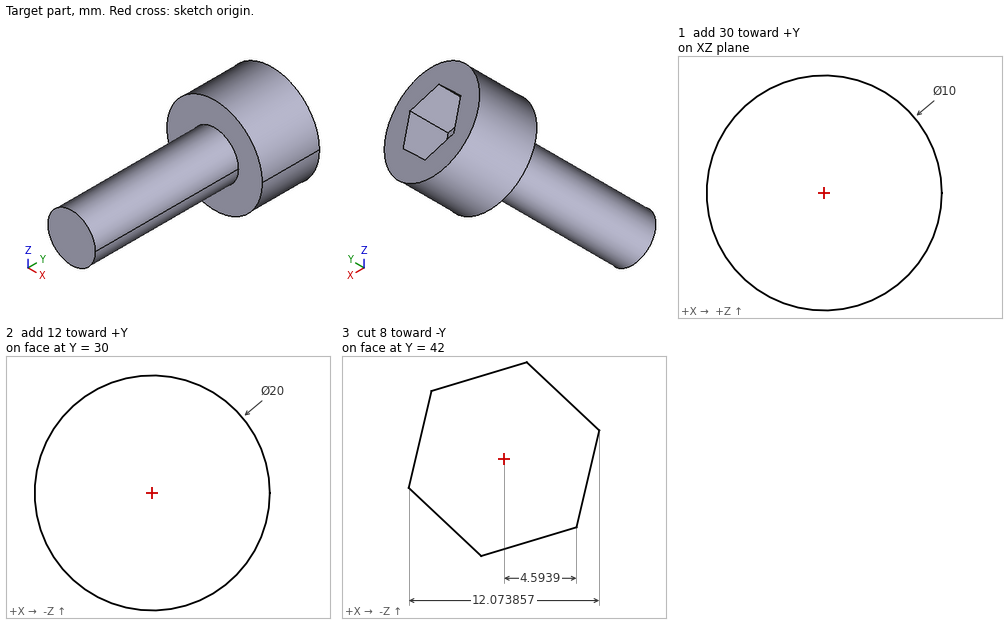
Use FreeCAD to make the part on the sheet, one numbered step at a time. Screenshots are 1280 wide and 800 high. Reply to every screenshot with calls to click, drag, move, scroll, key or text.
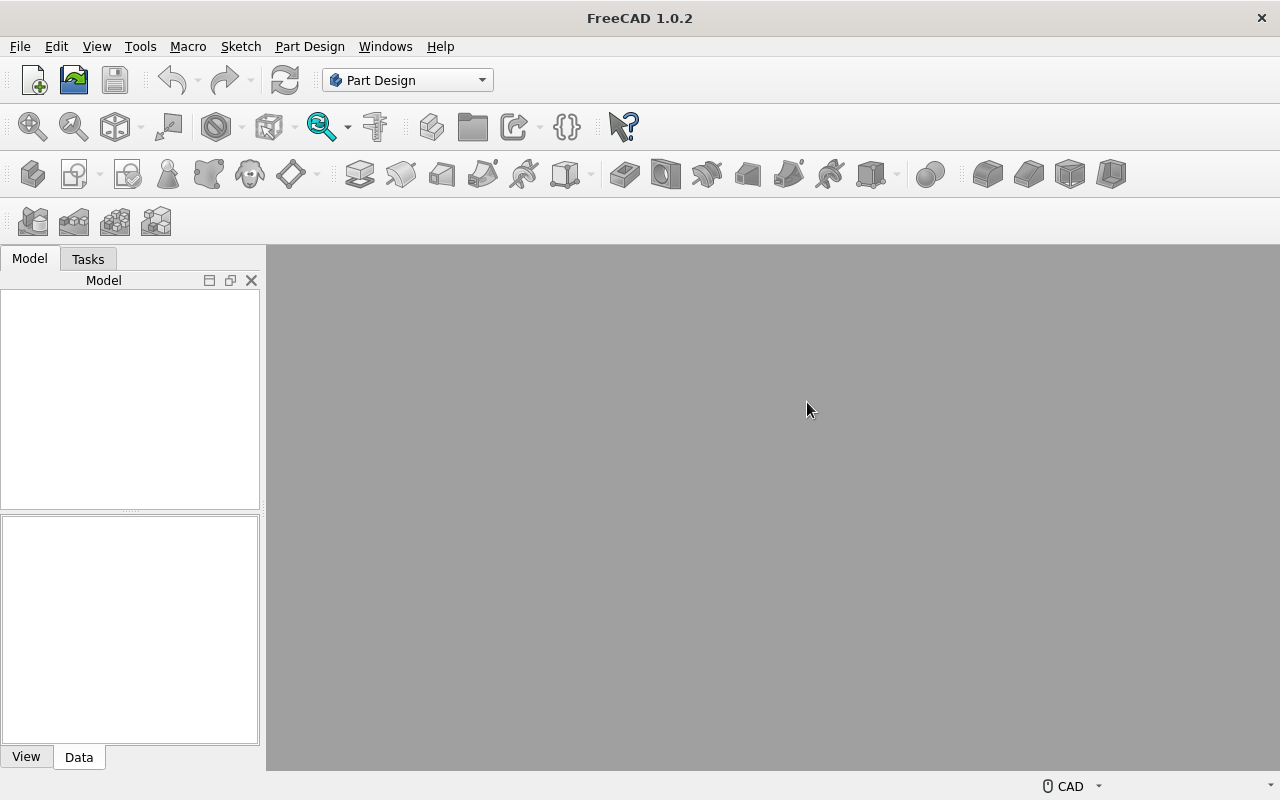
click(33, 80)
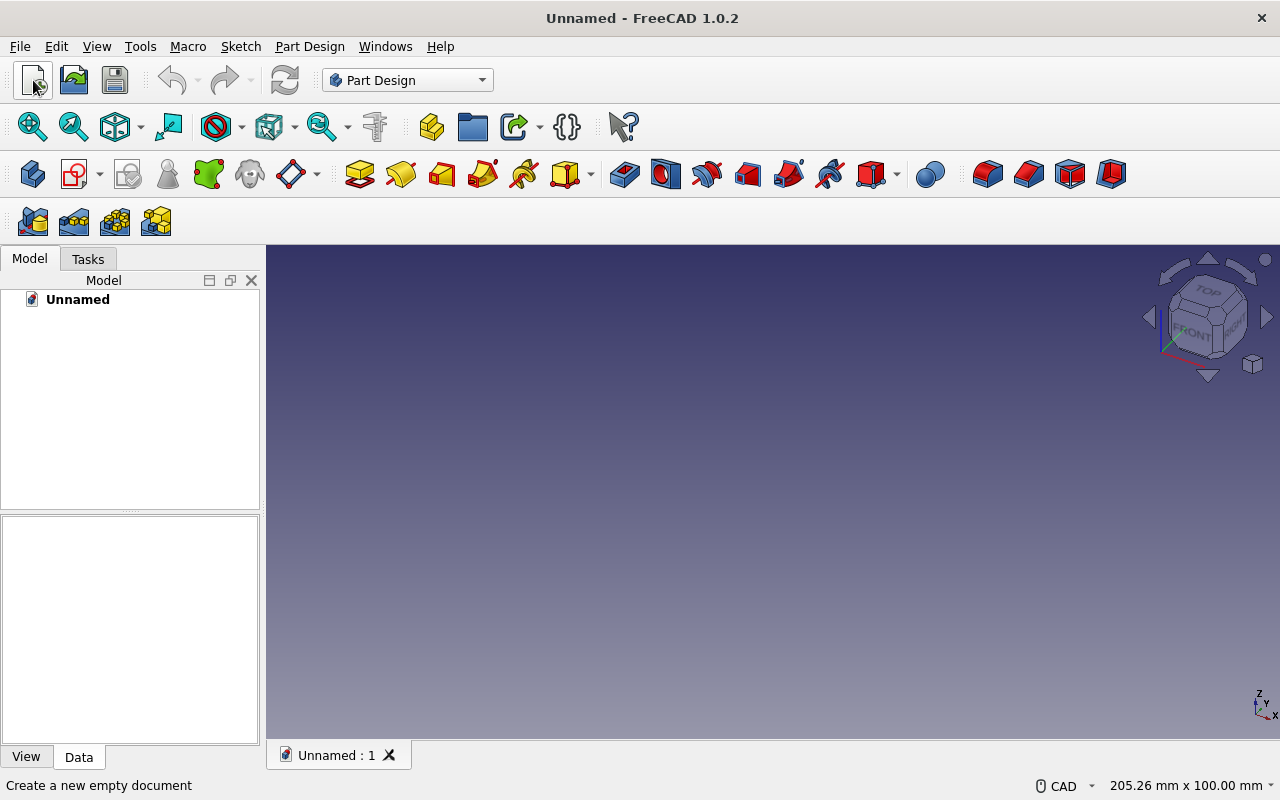
click(74, 174)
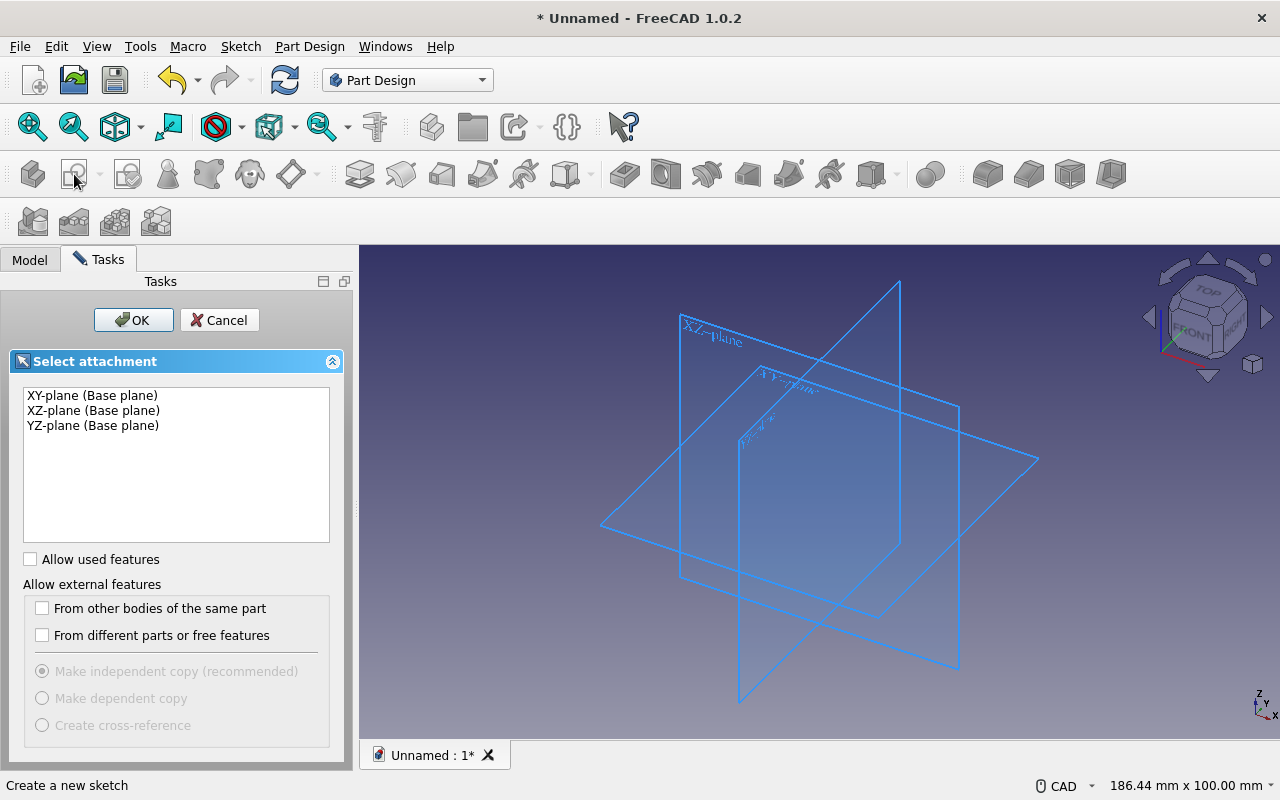
click(84, 410)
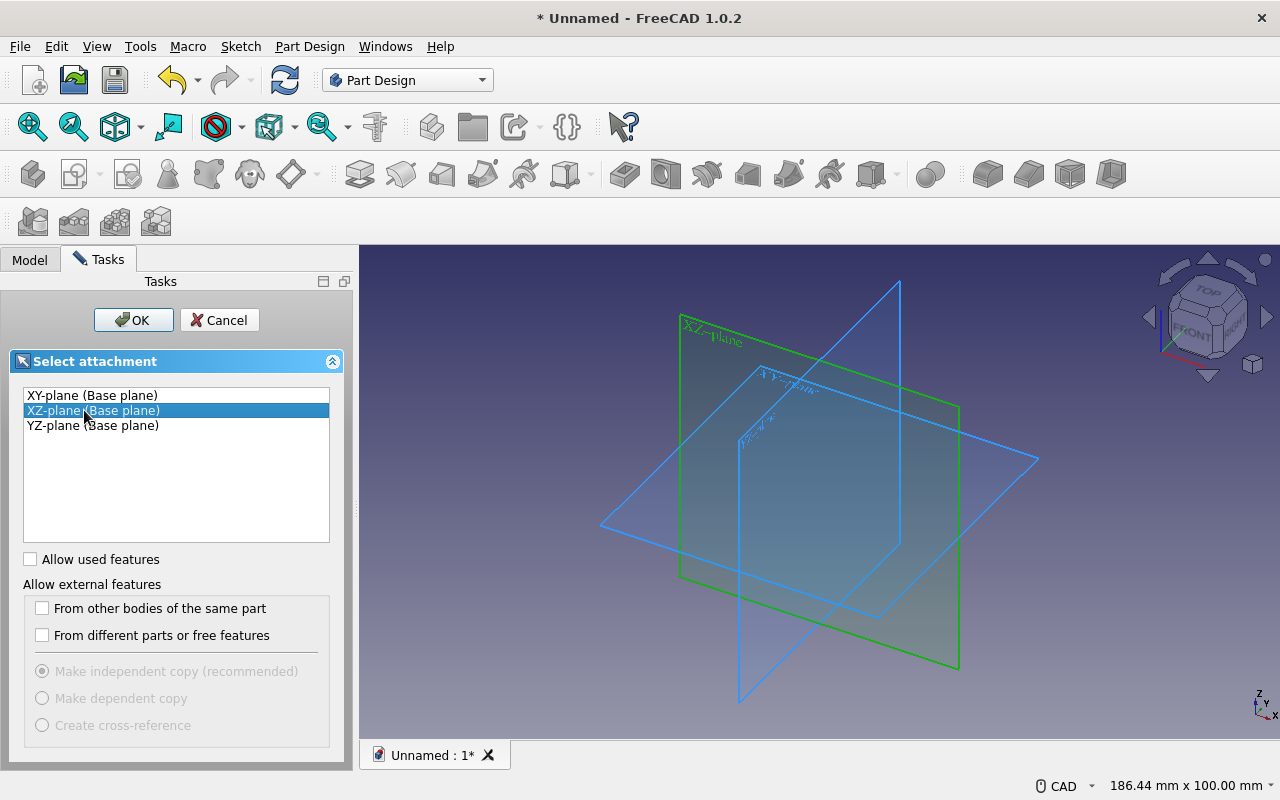
click(134, 320)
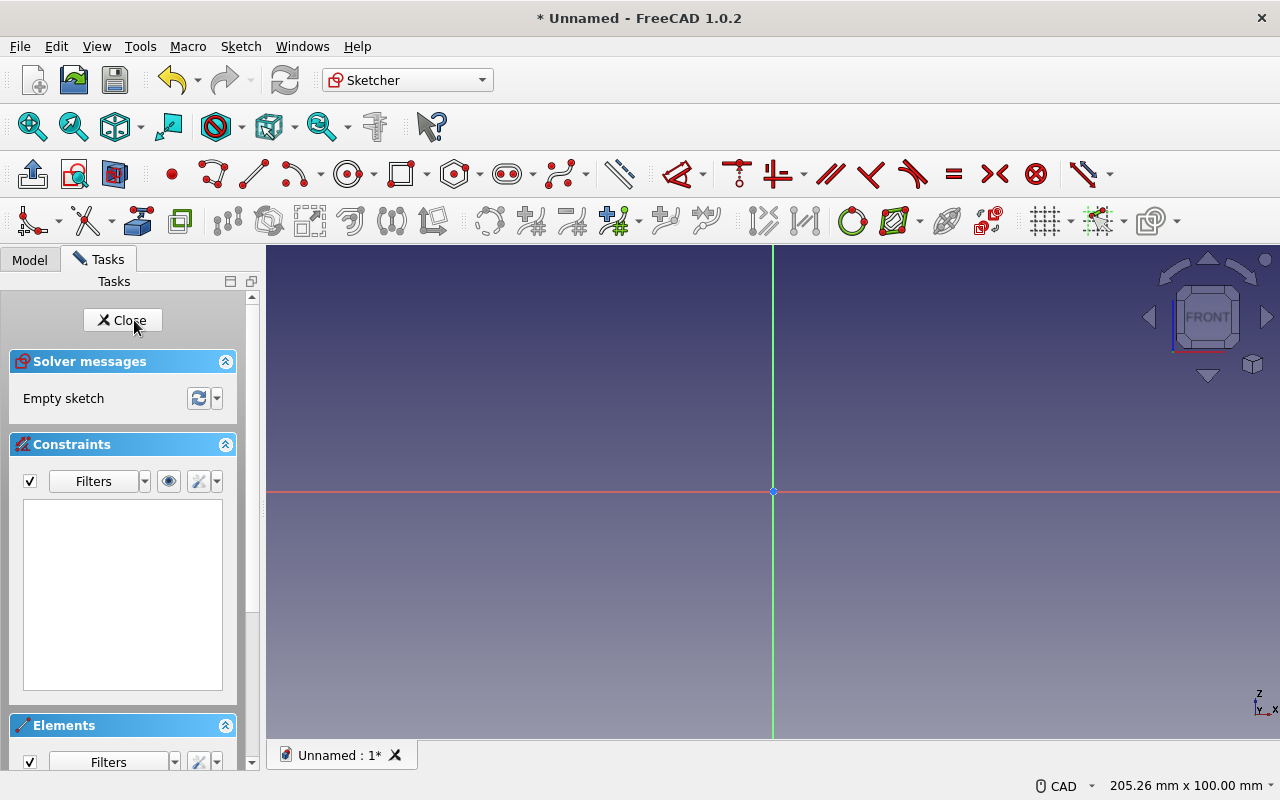
scroll(787, 492, up, 9)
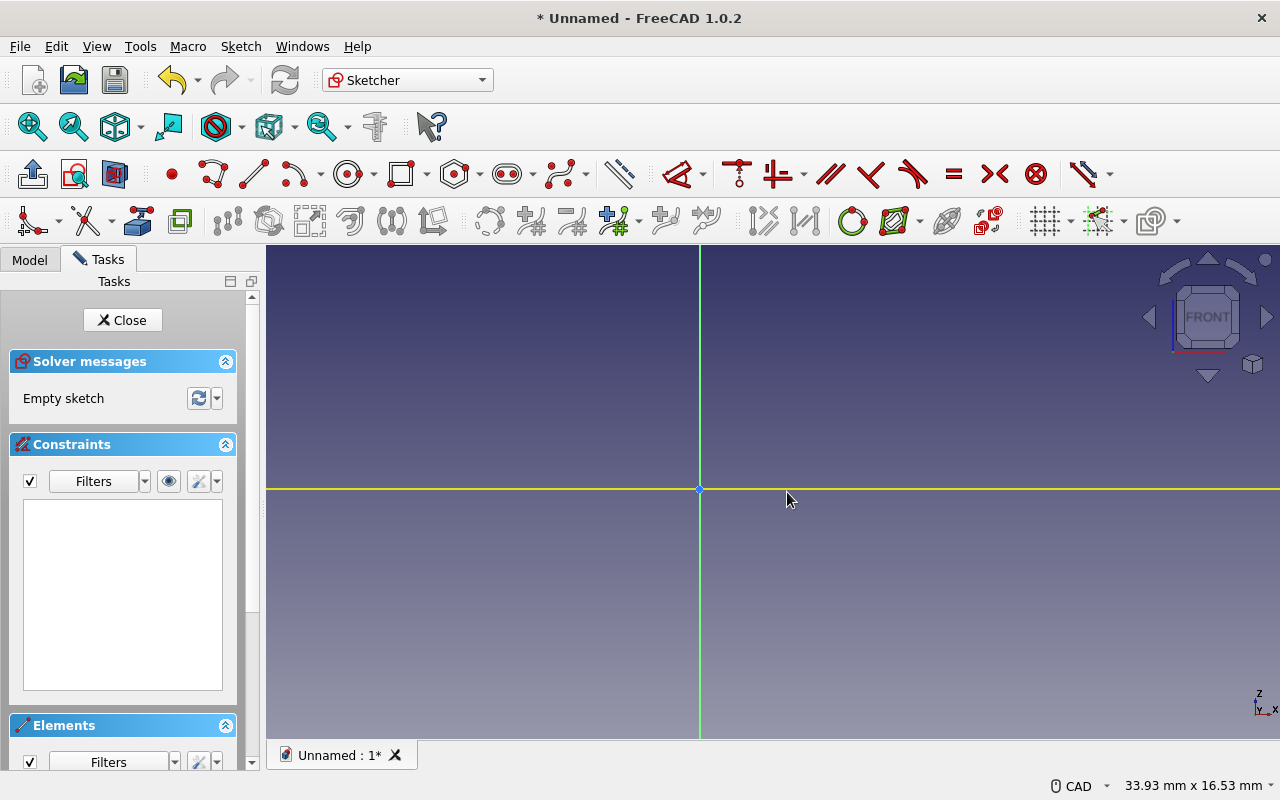
click(348, 174)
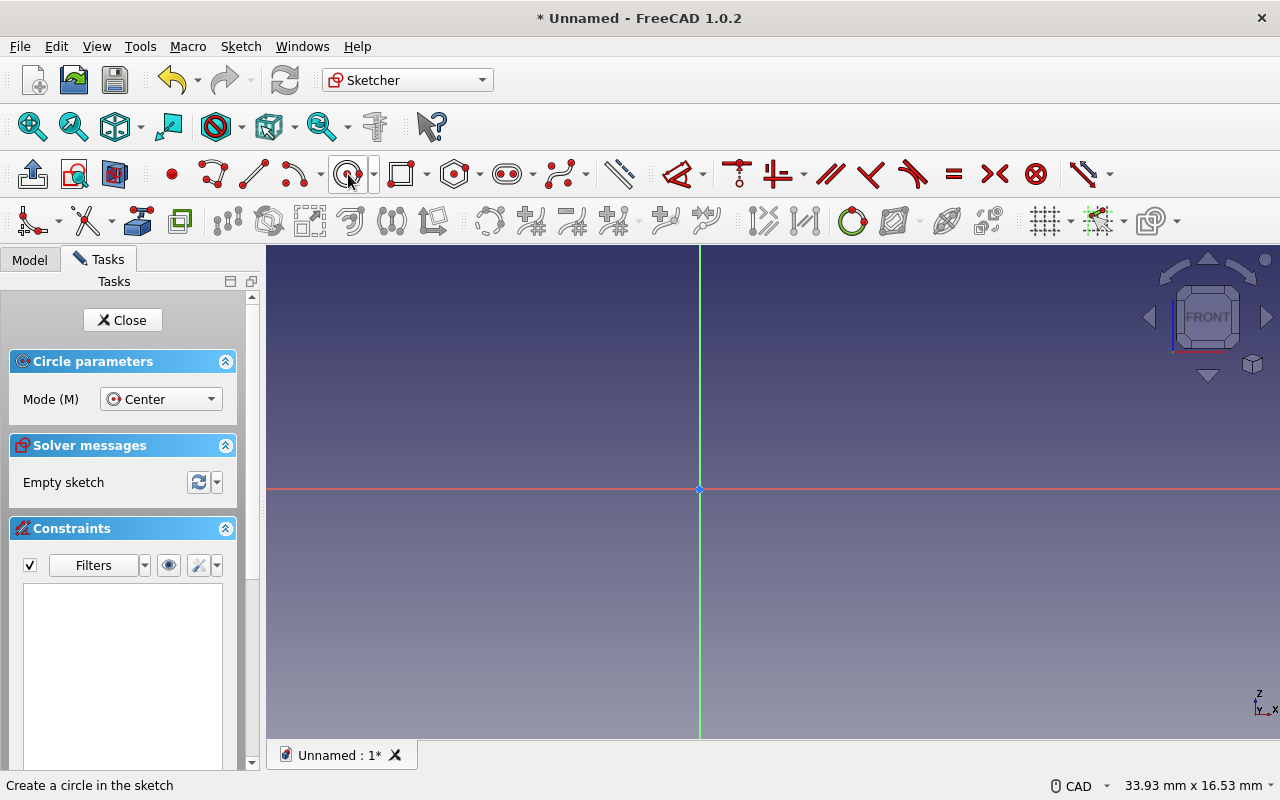
click(700, 489)
move(805, 384)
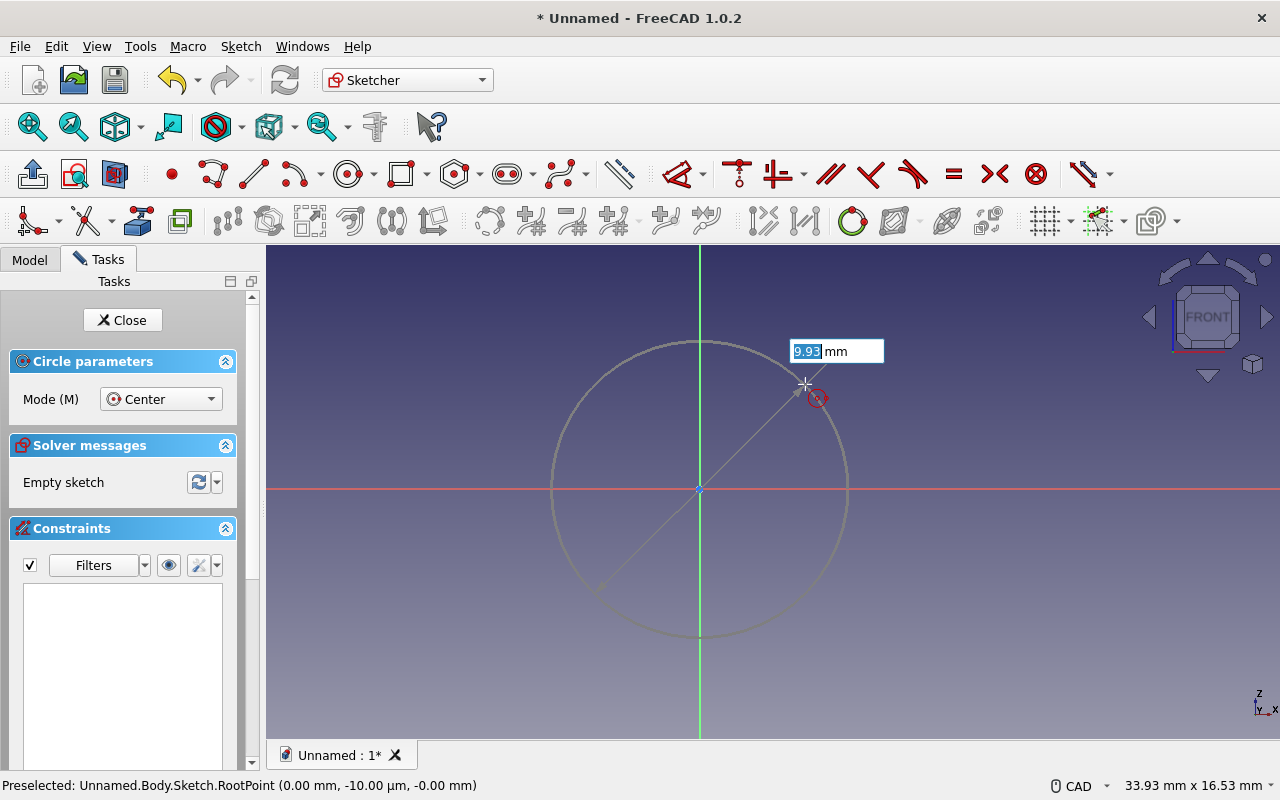
text(10)
key(Return)
key(Escape)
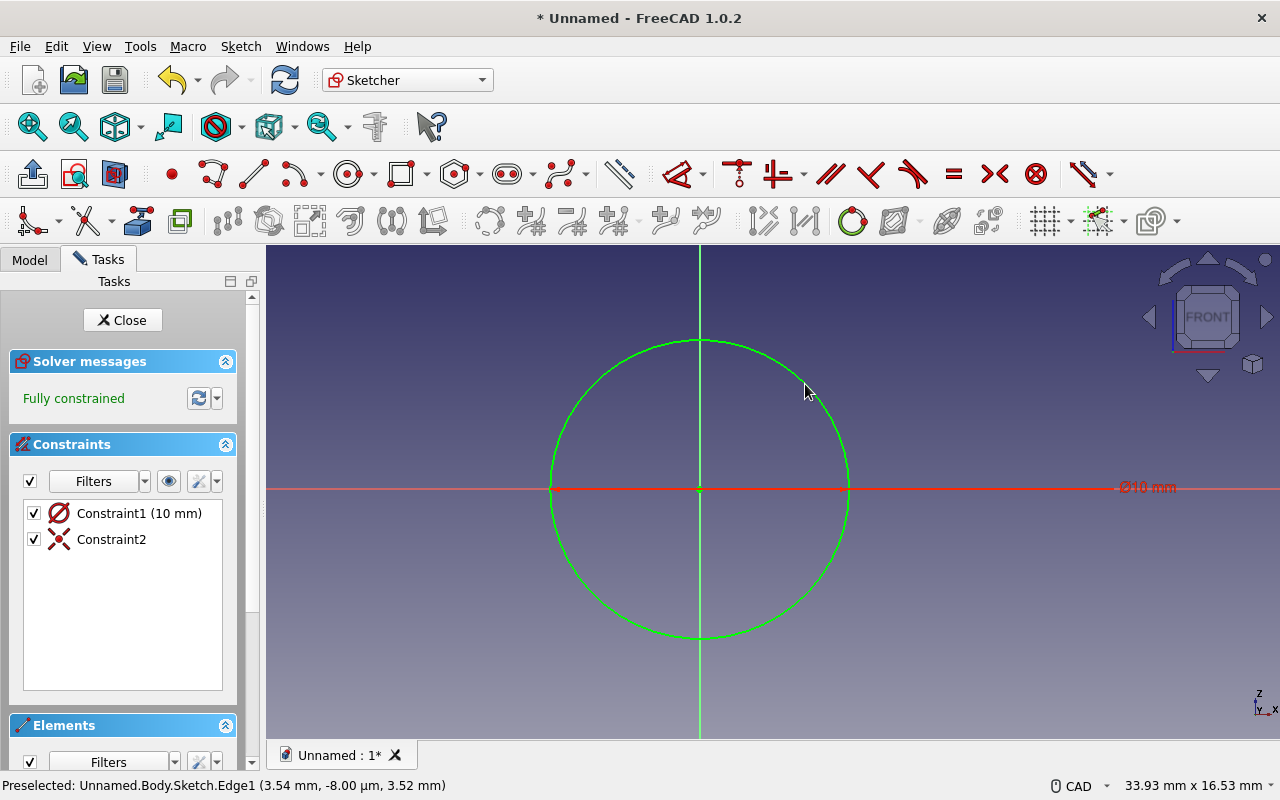
click(123, 320)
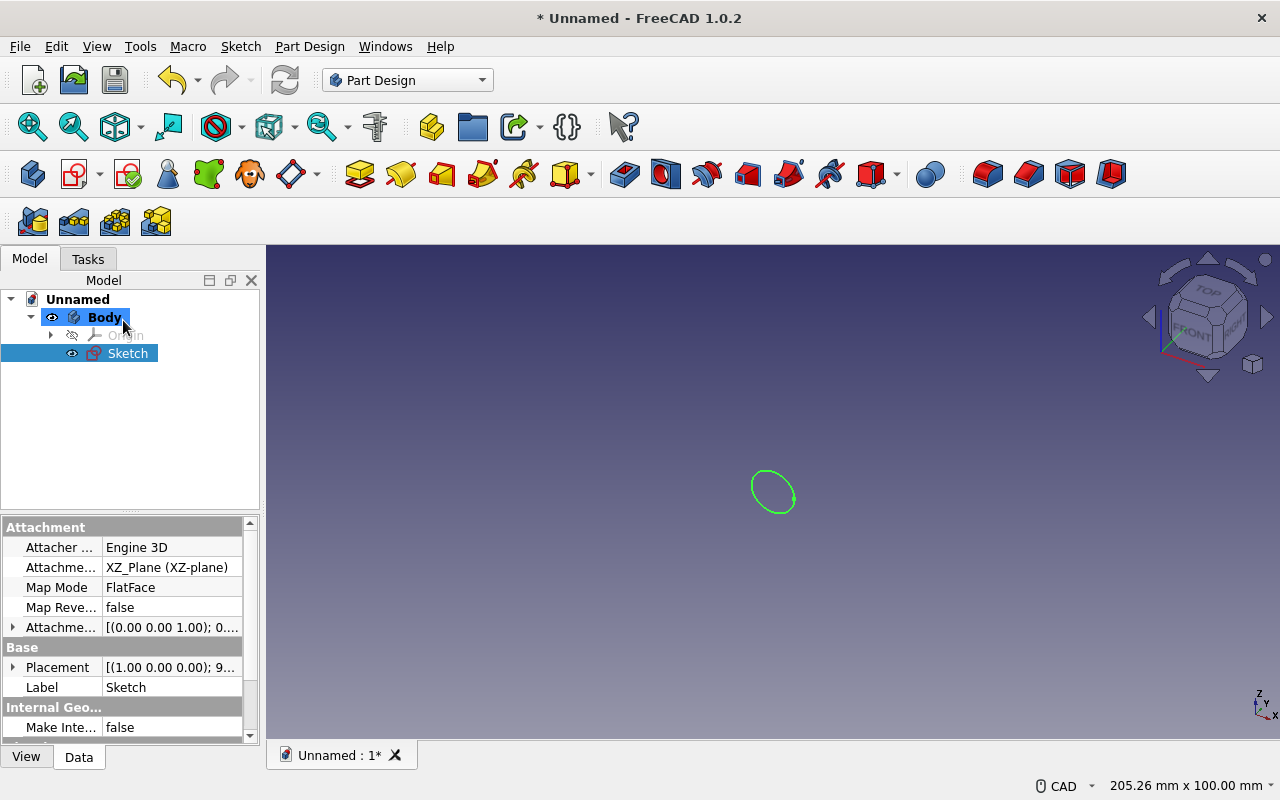
click(360, 174)